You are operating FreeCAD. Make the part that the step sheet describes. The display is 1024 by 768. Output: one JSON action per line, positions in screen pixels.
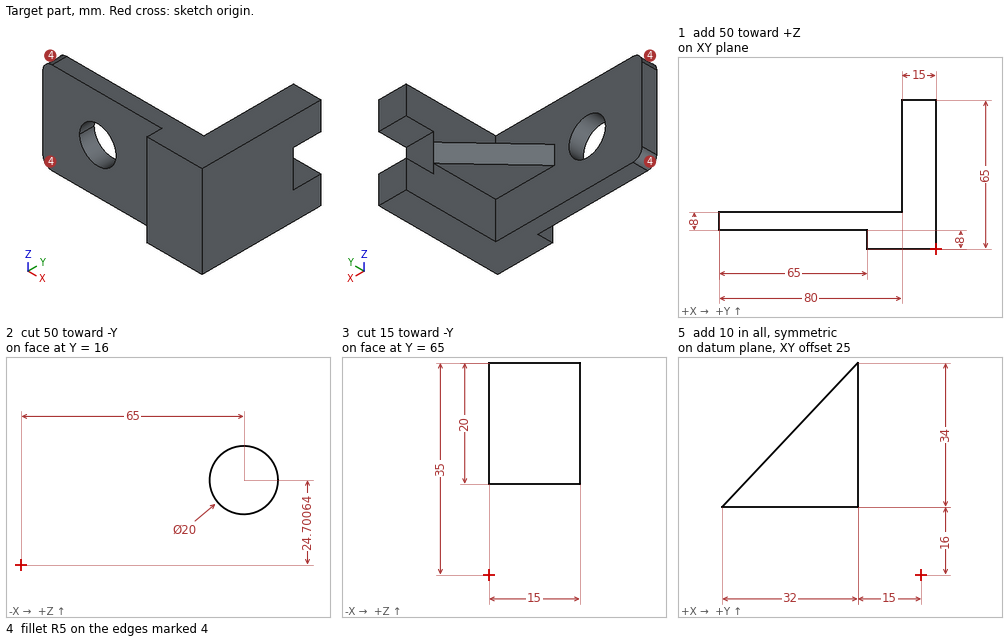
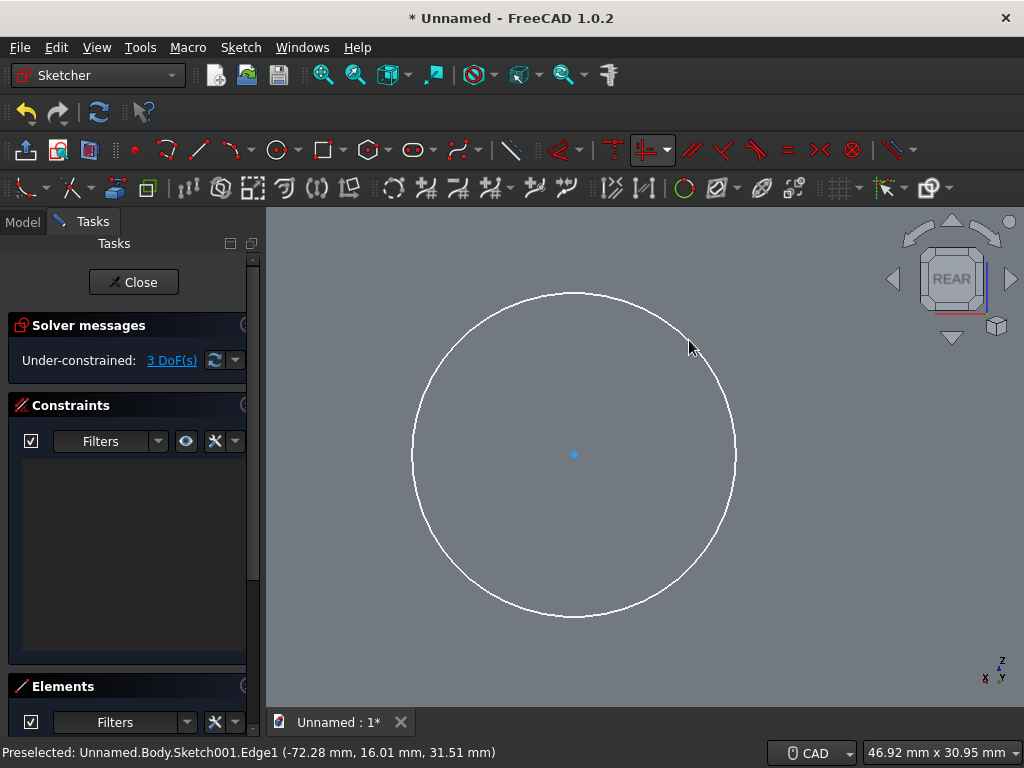
{"action": "key", "text": "d"}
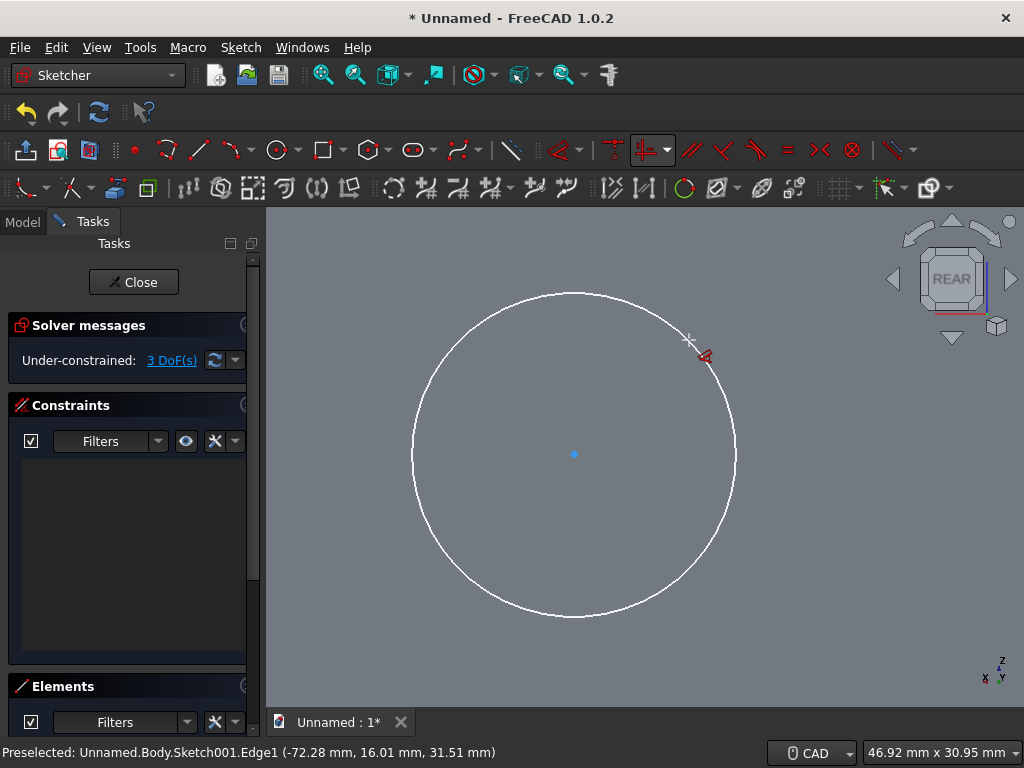
{"action": "left_click", "coordinate": [688, 340]}
{"action": "left_click", "coordinate": [711, 317]}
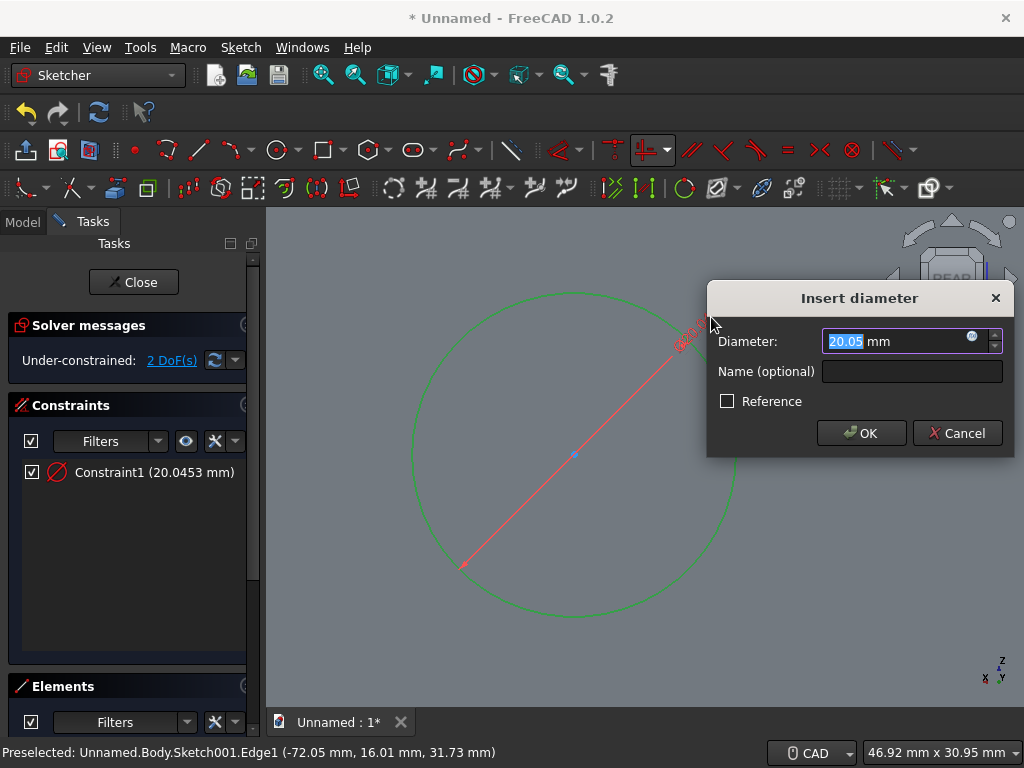
{"action": "type", "text": "20"}
{"action": "key", "text": "Return"}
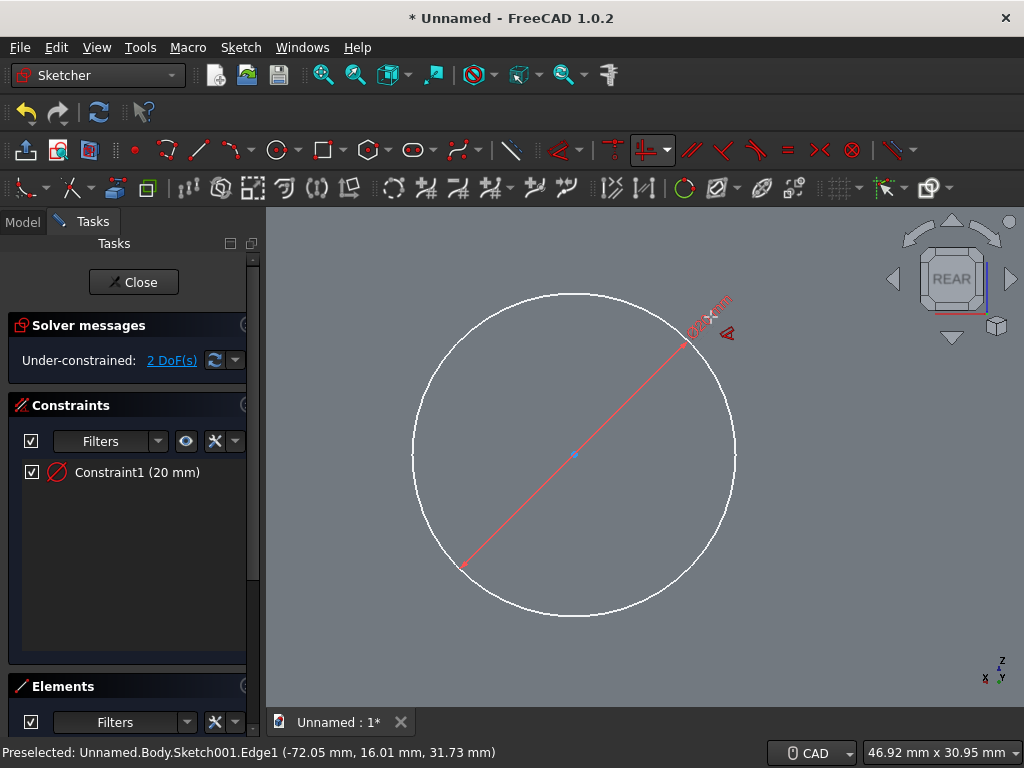
{"action": "left_click", "coordinate": [574, 455]}
{"action": "left_click", "coordinate": [434, 421]}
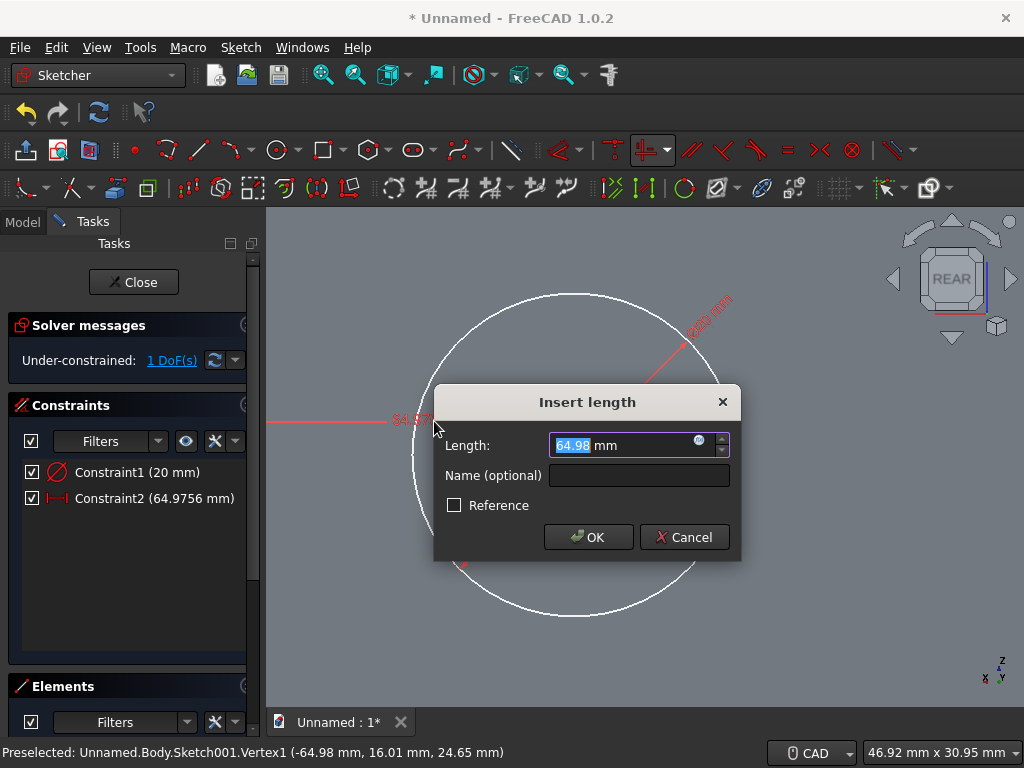
{"action": "type", "text": "65"}
{"action": "key", "text": "Return"}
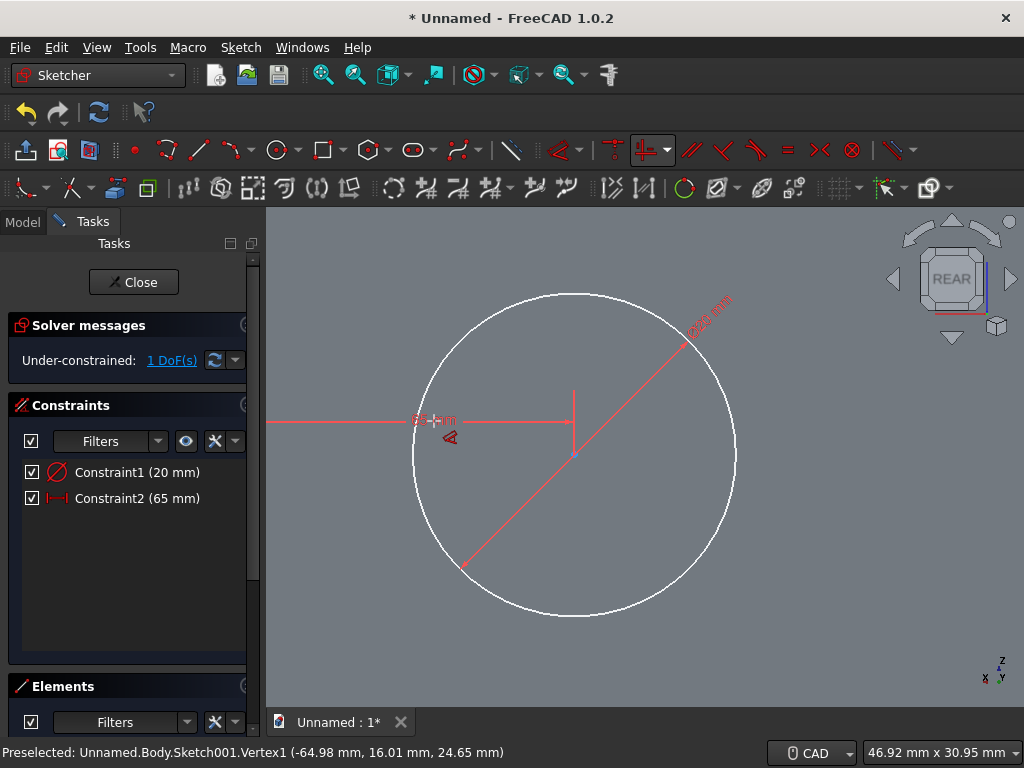
{"action": "left_click", "coordinate": [574, 455]}
{"action": "left_click", "coordinate": [608, 567]}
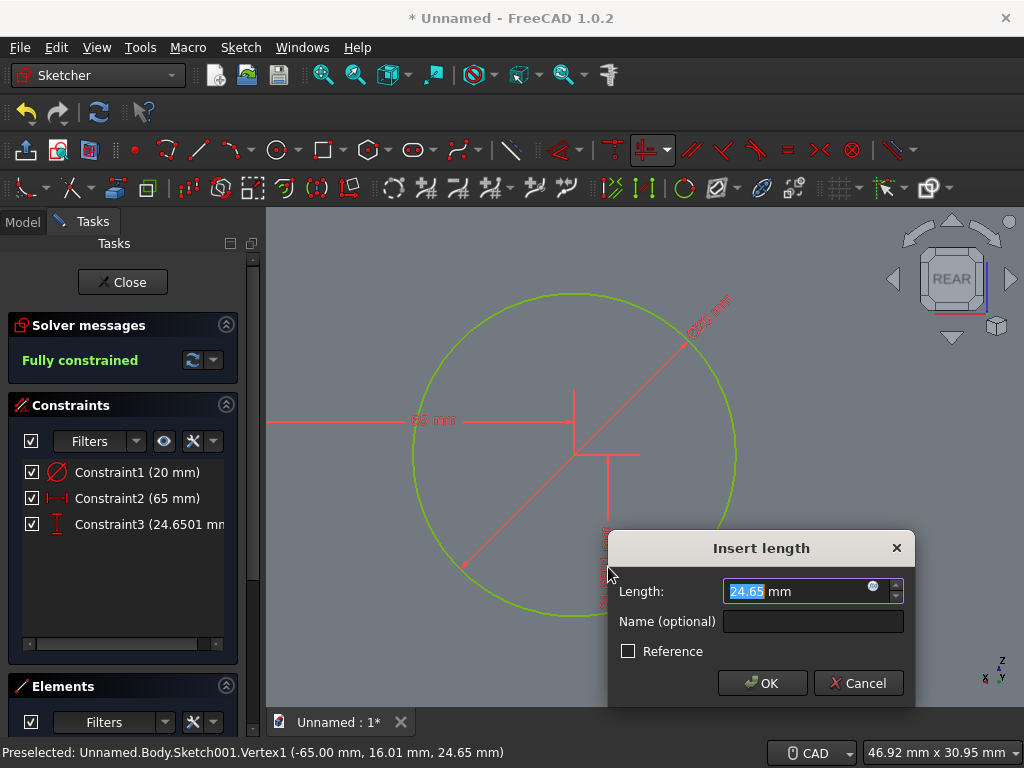
{"action": "type", "text": "24.70064"}
{"action": "key", "text": "Return"}
{"action": "key", "text": "Escape"}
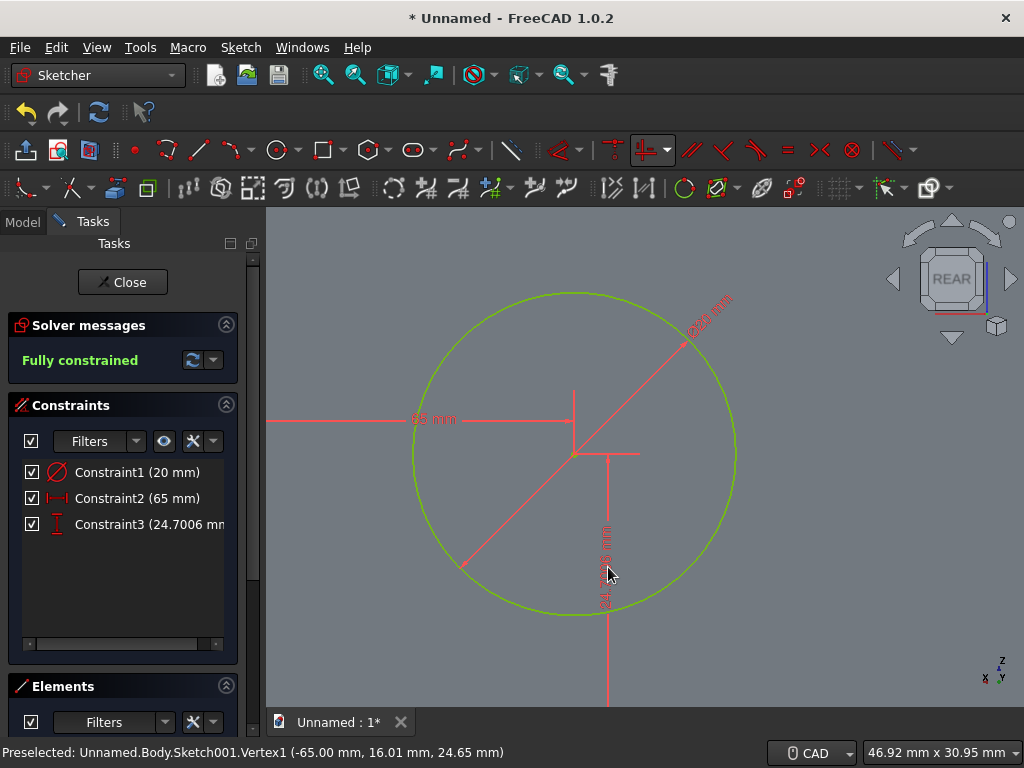
{"action": "left_click", "coordinate": [123, 282]}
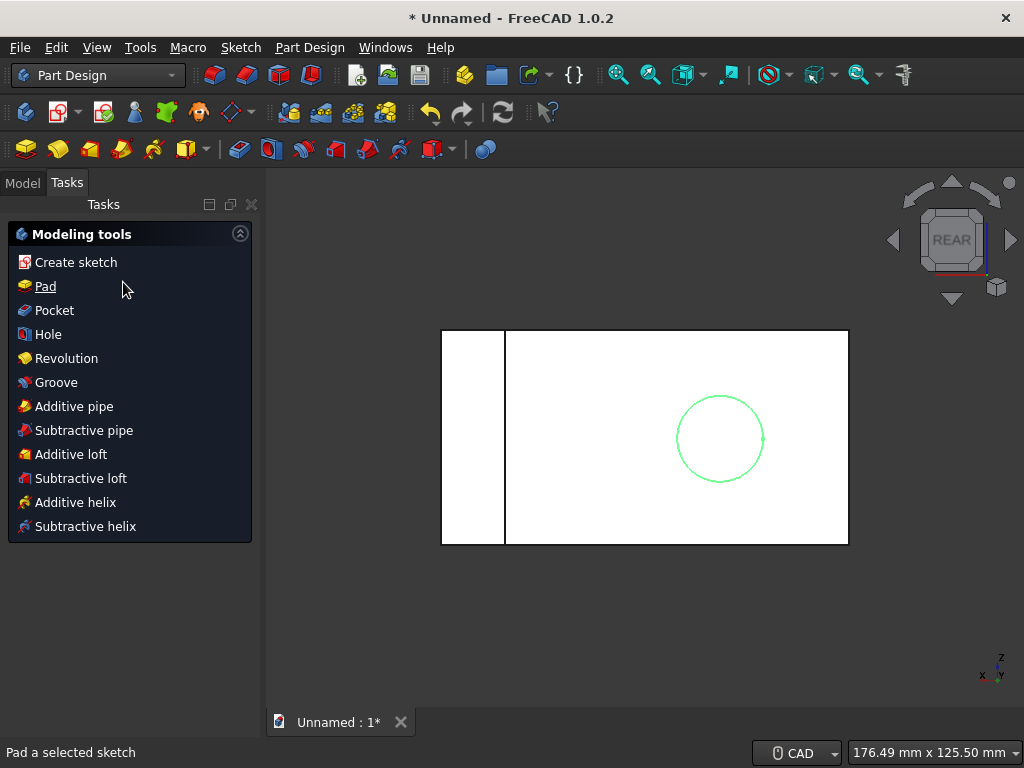
{"action": "left_click", "coordinate": [240, 150]}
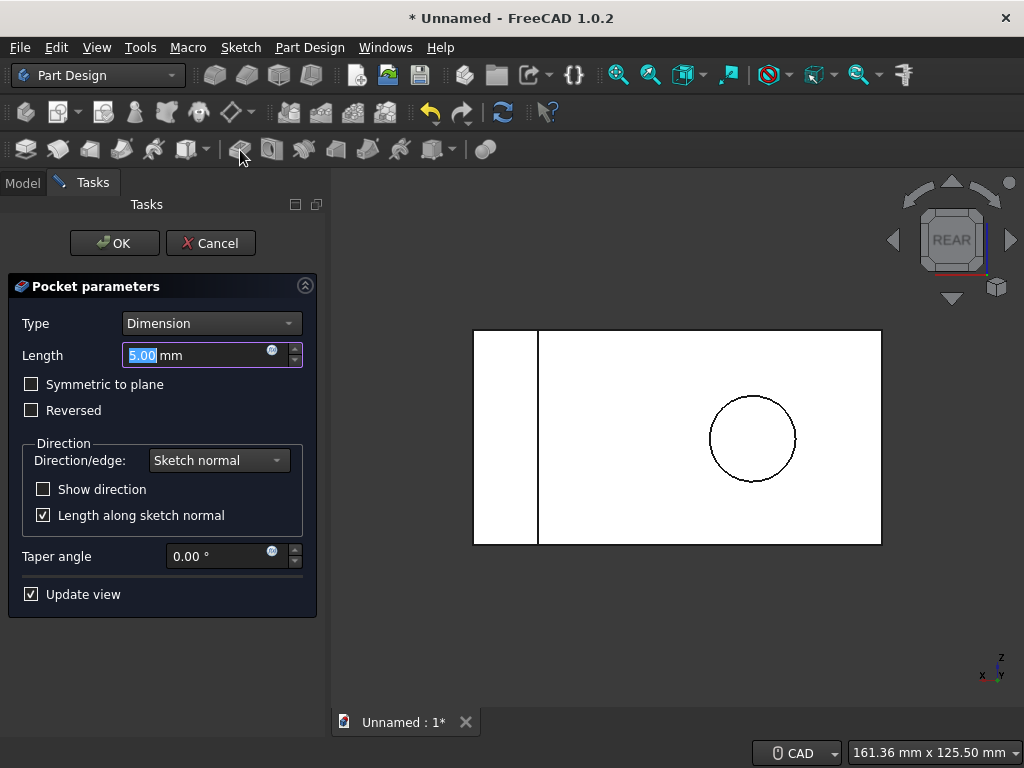
{"action": "type", "text": "50"}
{"action": "key", "text": "Tab"}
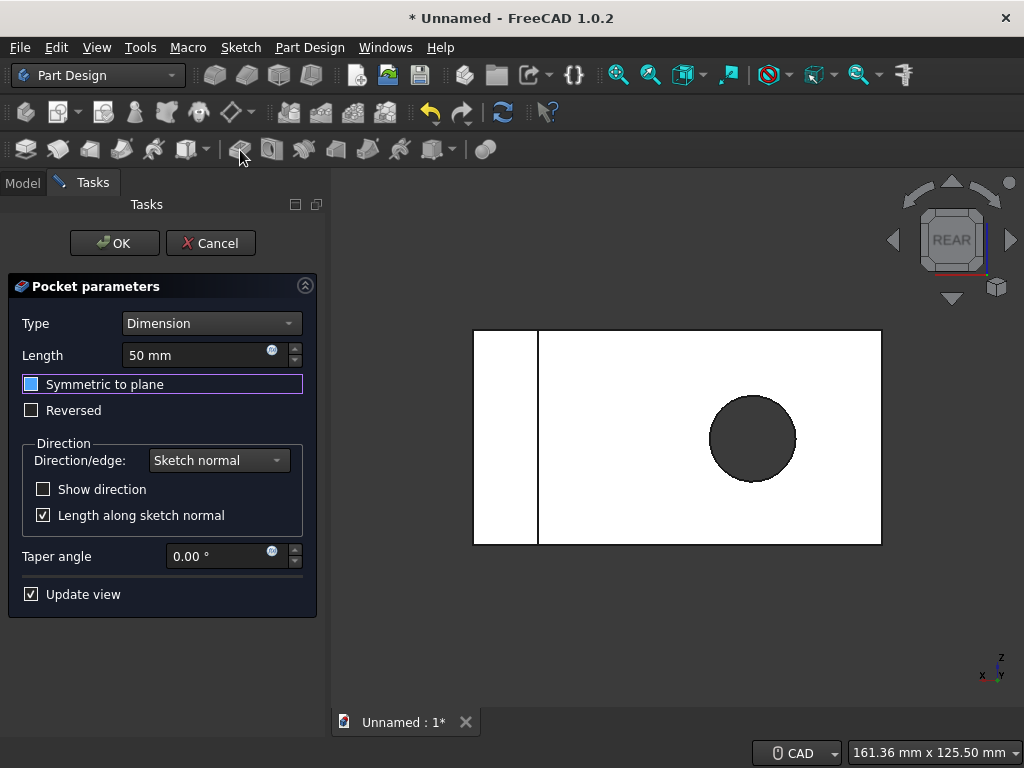
{"action": "left_click", "coordinate": [115, 243]}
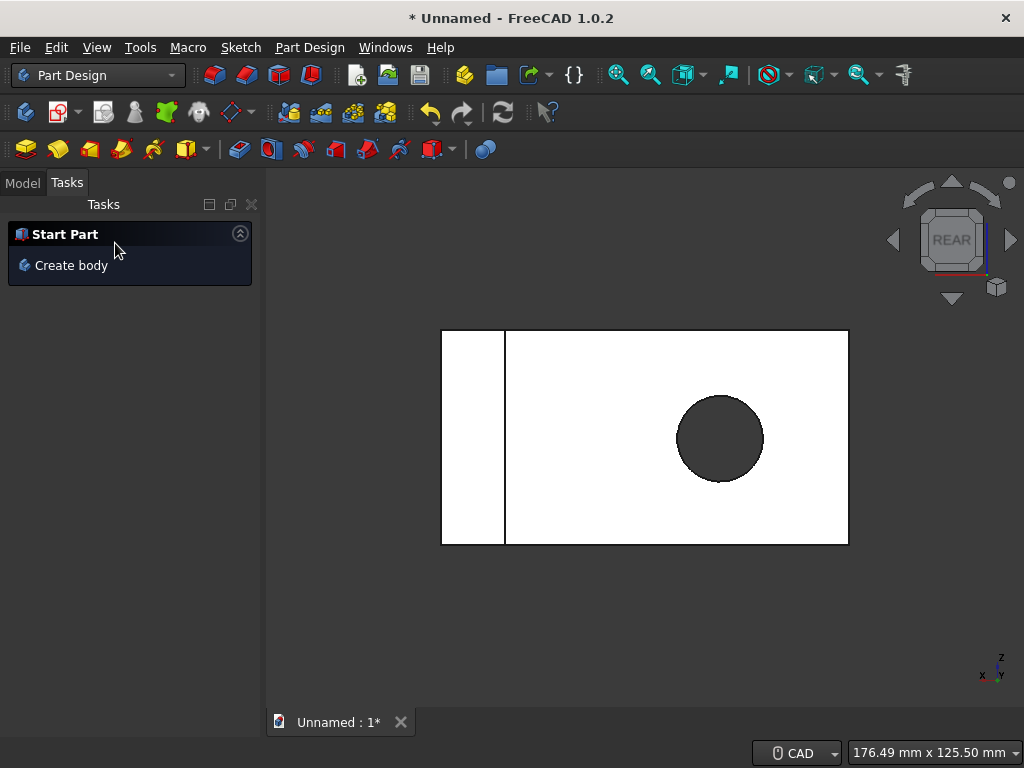
{"action": "left_click", "coordinate": [473, 375]}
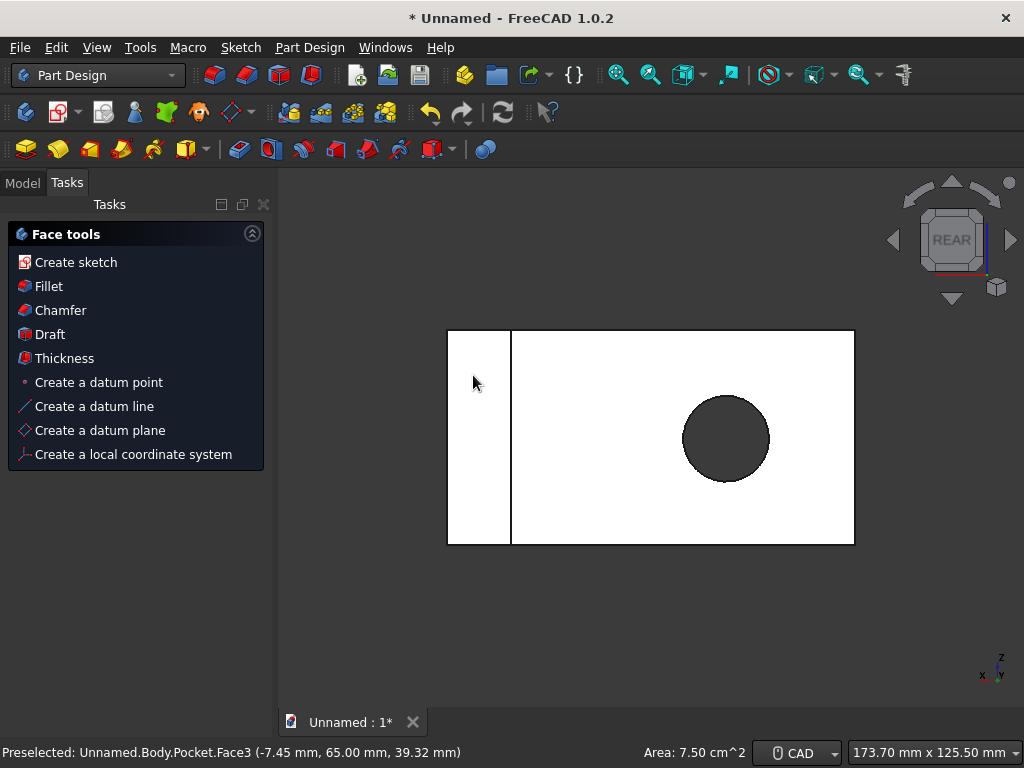
{"action": "left_click", "coordinate": [58, 112]}